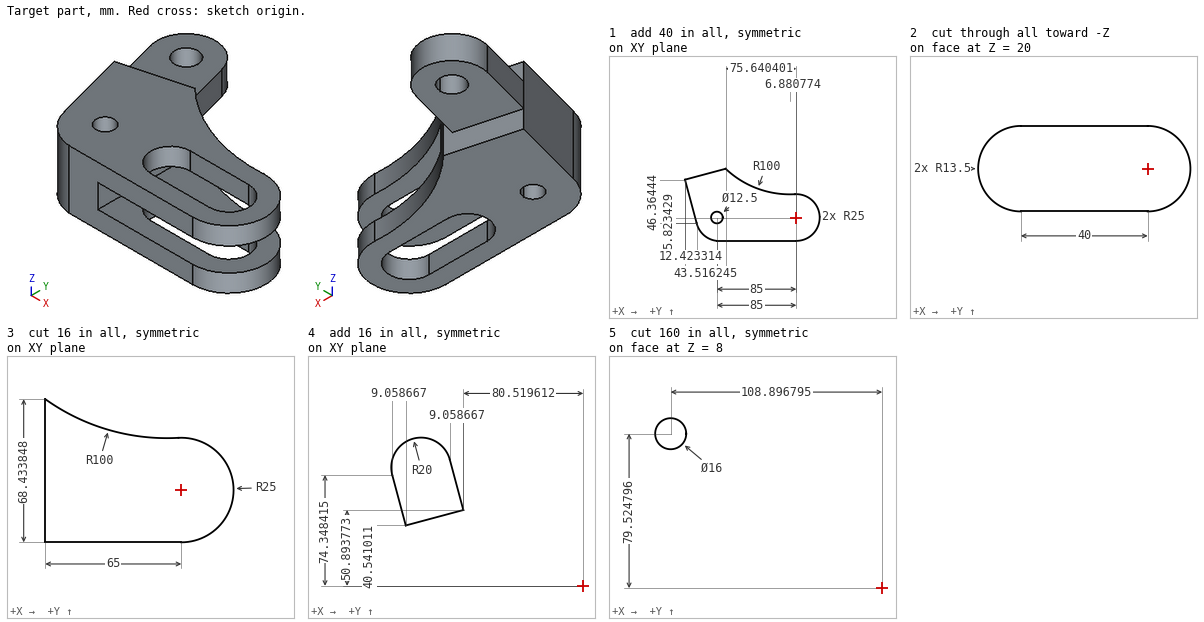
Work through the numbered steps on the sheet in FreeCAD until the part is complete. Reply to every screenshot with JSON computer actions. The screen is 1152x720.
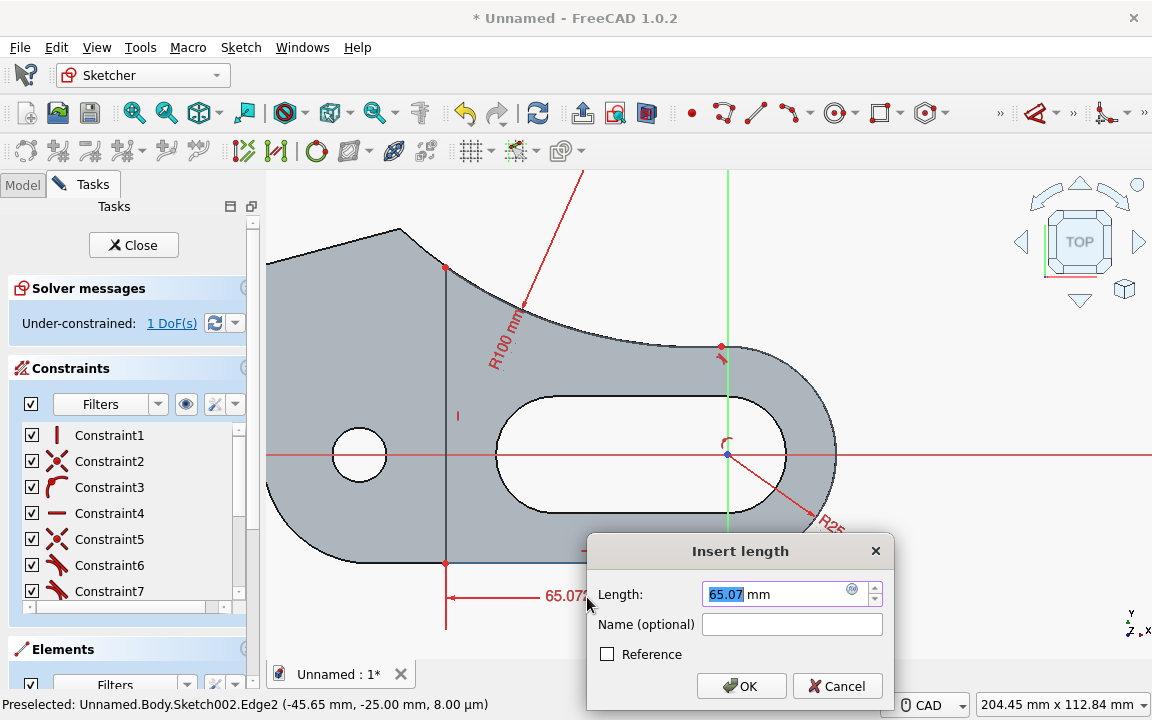
{"action": "type", "text": "65"}
{"action": "key", "text": "Return"}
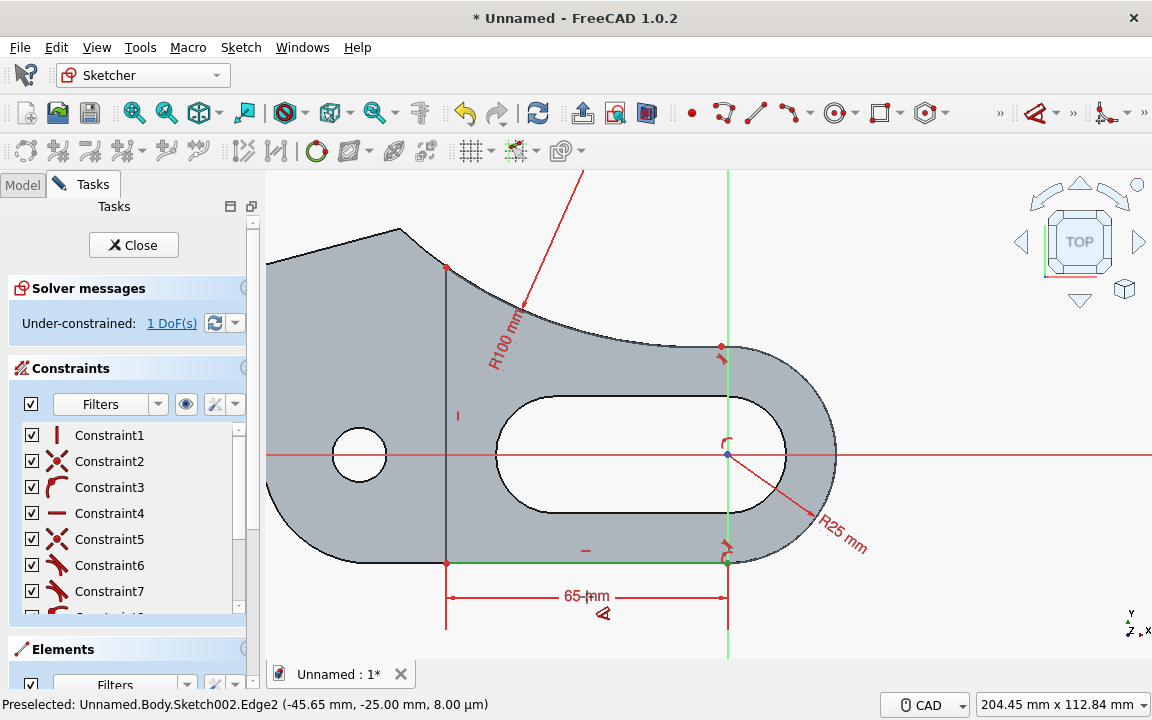
{"action": "left_click", "coordinate": [446, 356]}
{"action": "left_click", "coordinate": [412, 415]}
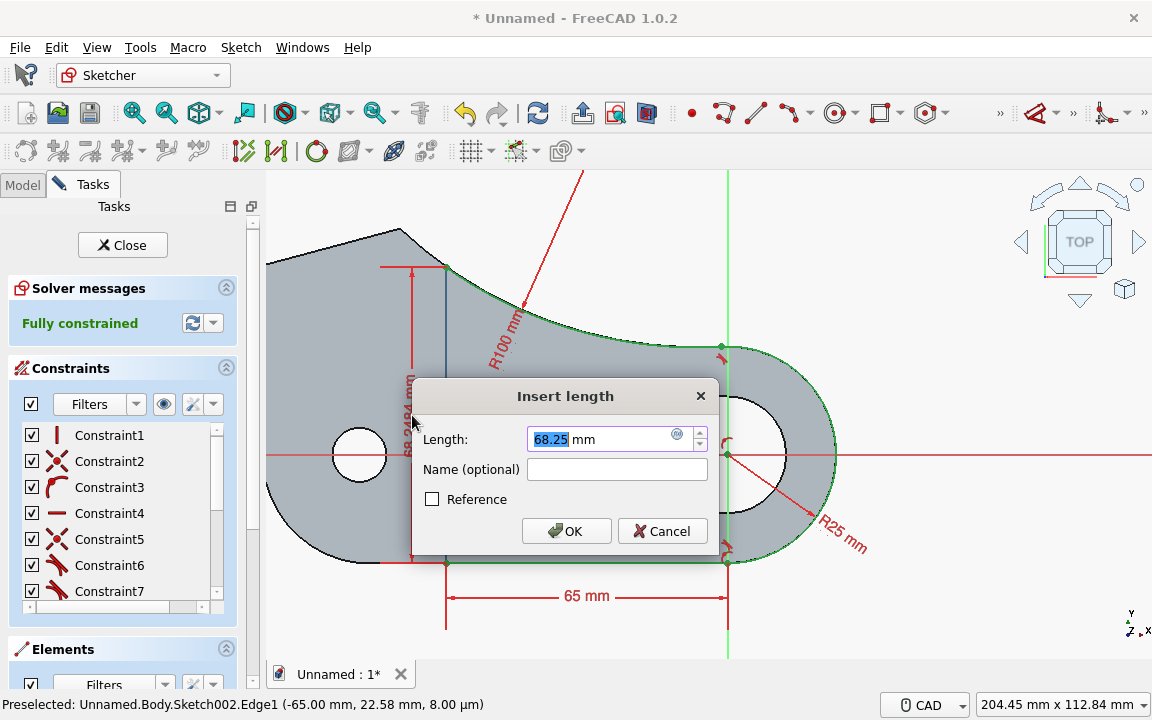
{"action": "type", "text": "68.433848"}
{"action": "key", "text": "Return"}
{"action": "key", "text": "Escape"}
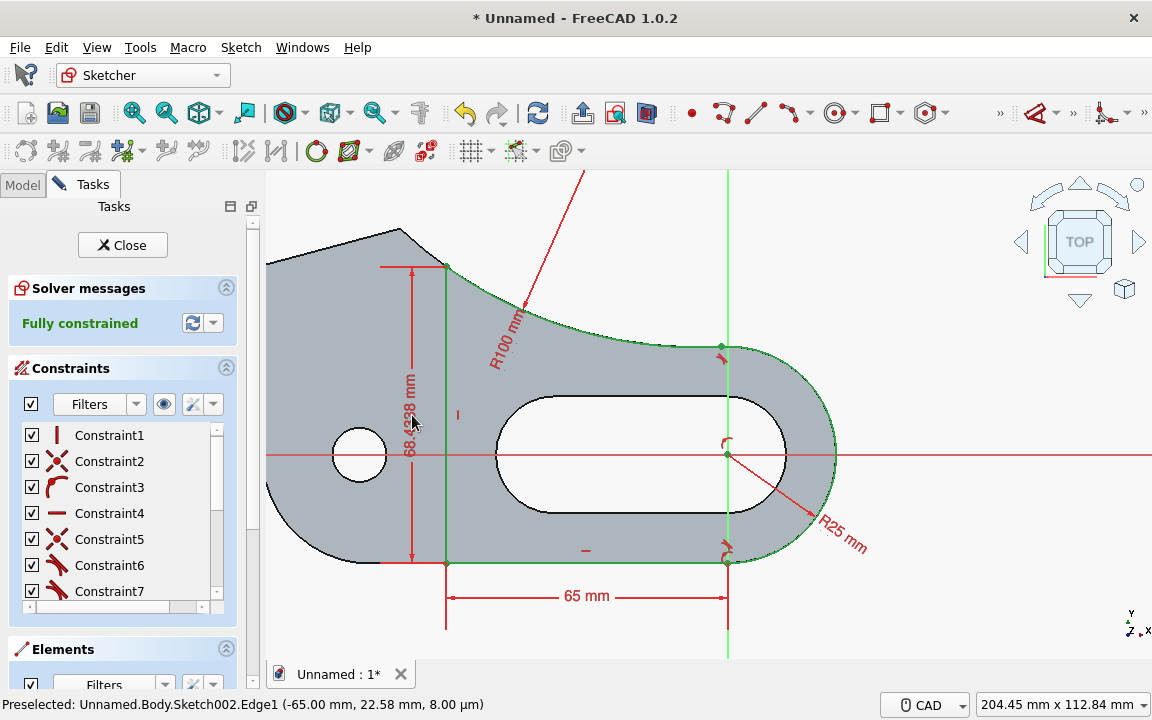
{"action": "left_click", "coordinate": [123, 245]}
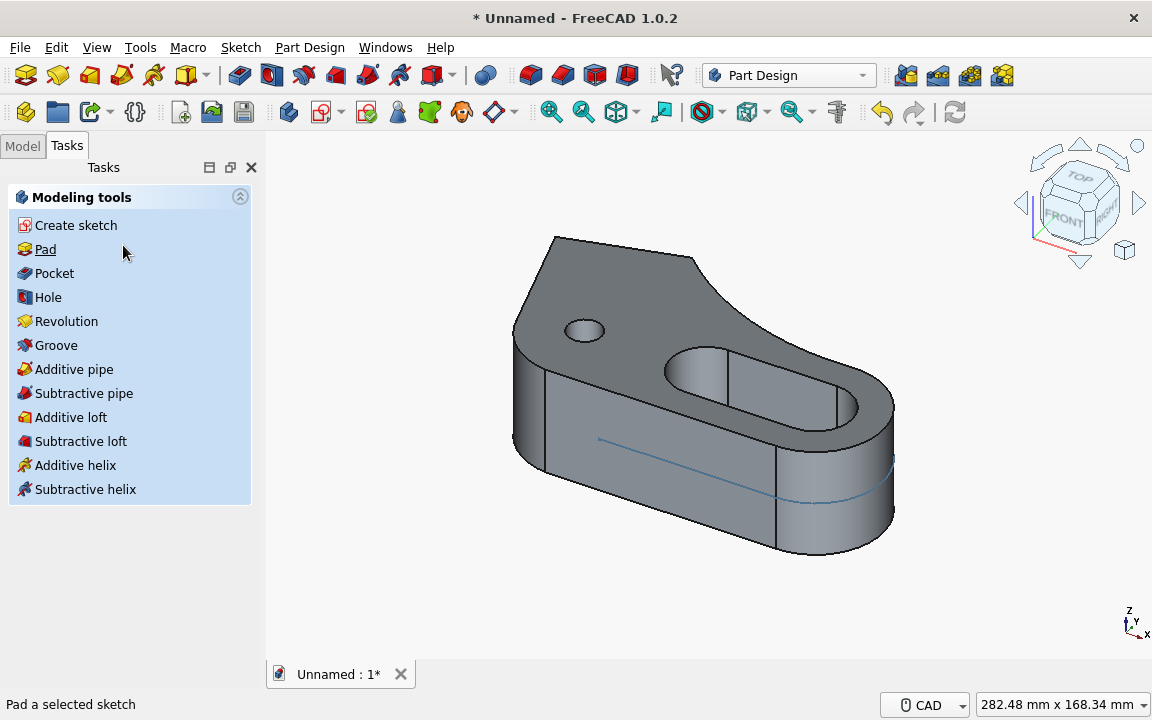
{"action": "left_click", "coordinate": [240, 76]}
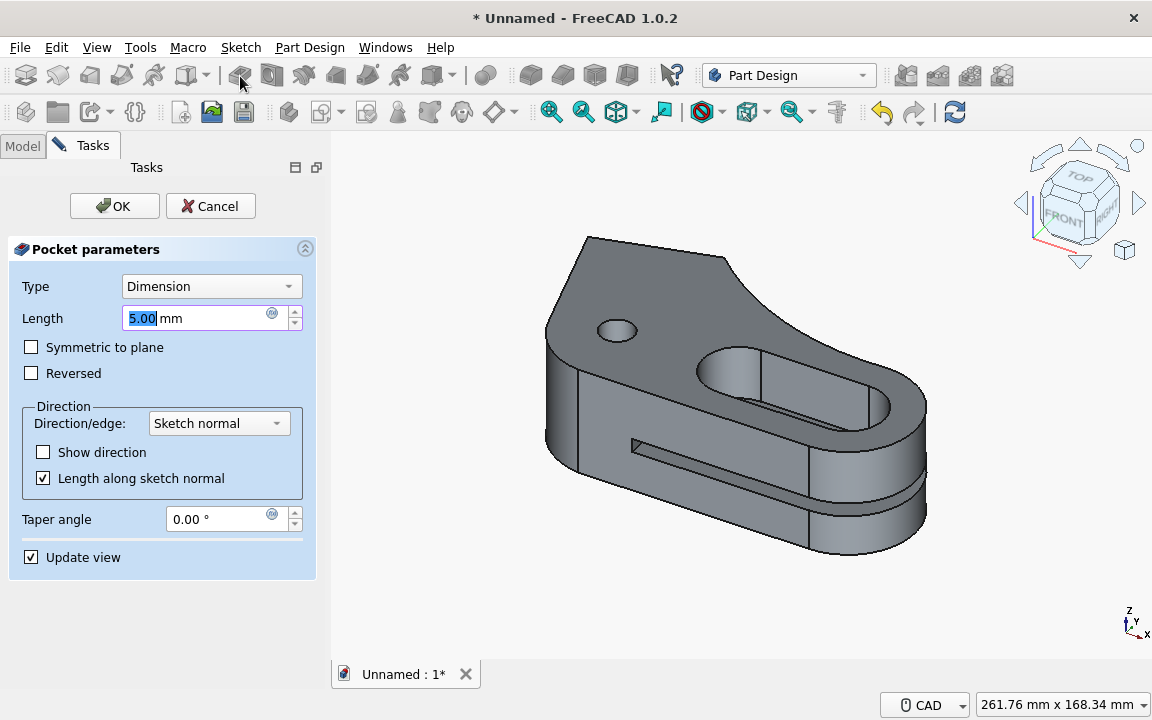
{"action": "type", "text": "16"}
{"action": "key", "text": "Tab"}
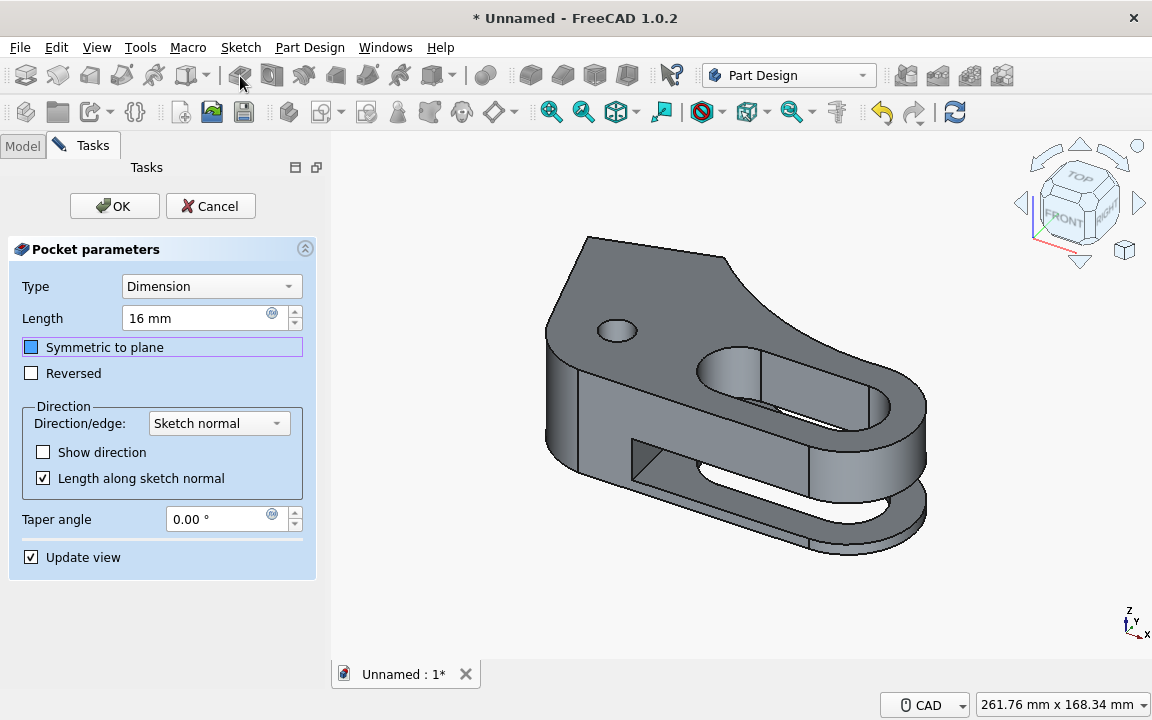
{"action": "left_click", "coordinate": [30, 347]}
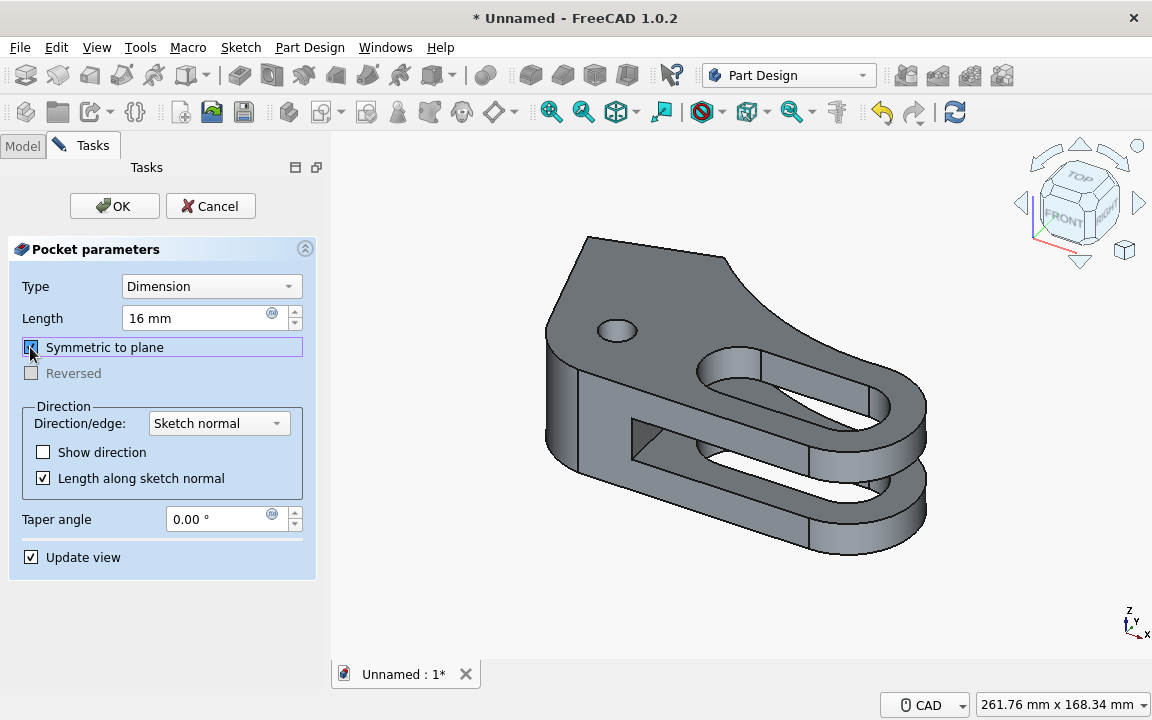
{"action": "left_click", "coordinate": [115, 206]}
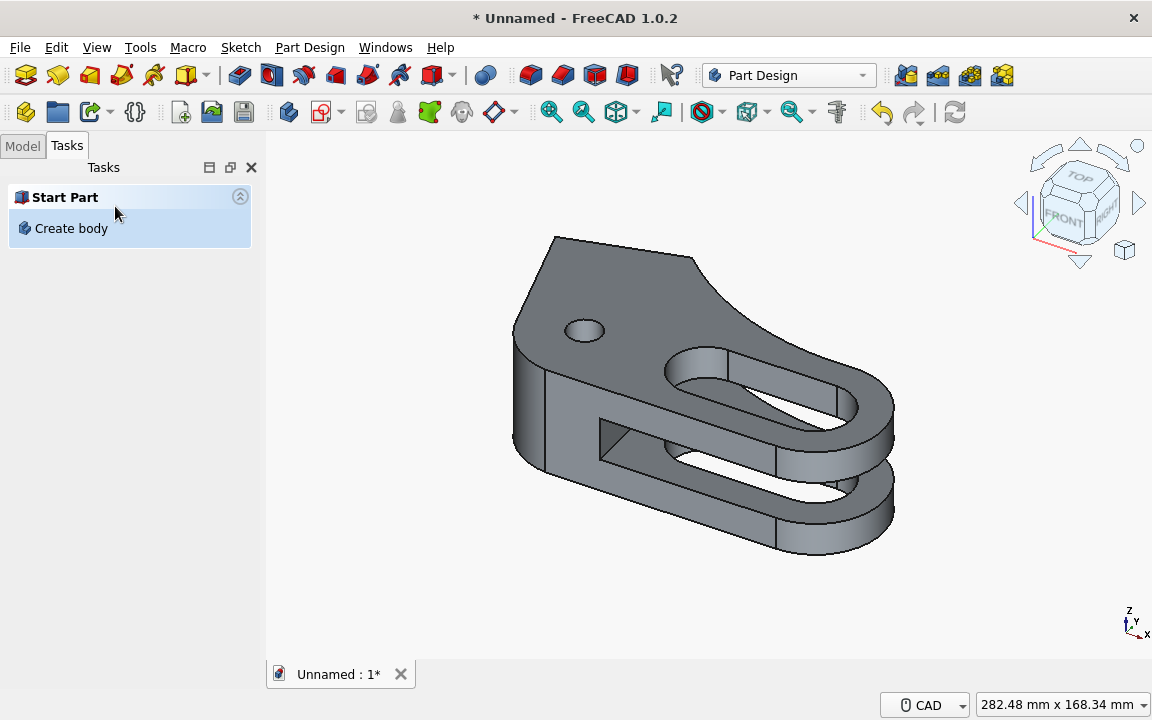
{"action": "left_click", "coordinate": [322, 112]}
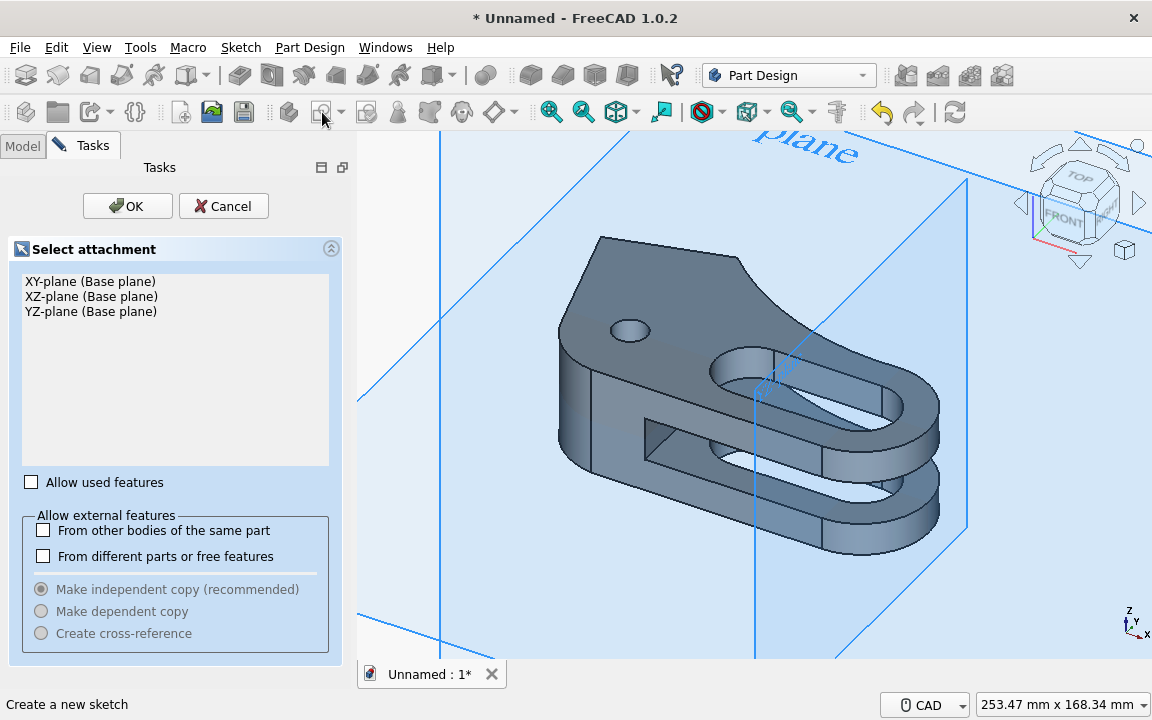
{"action": "left_click", "coordinate": [82, 282]}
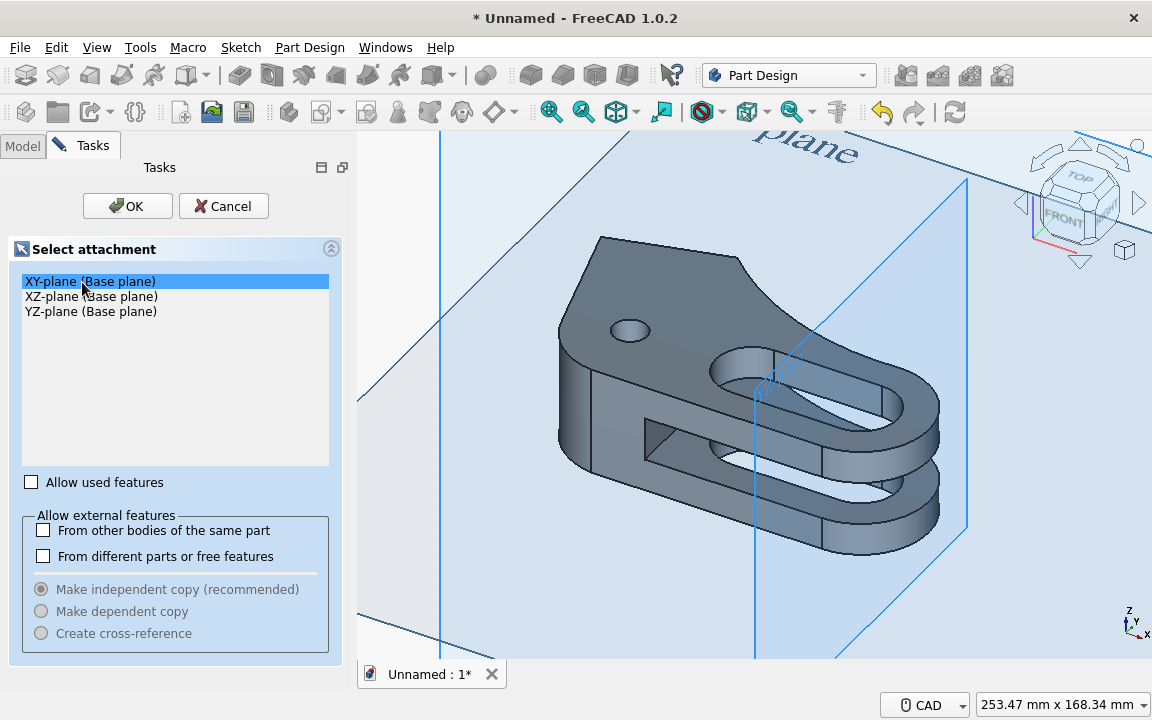
{"action": "left_click", "coordinate": [128, 206]}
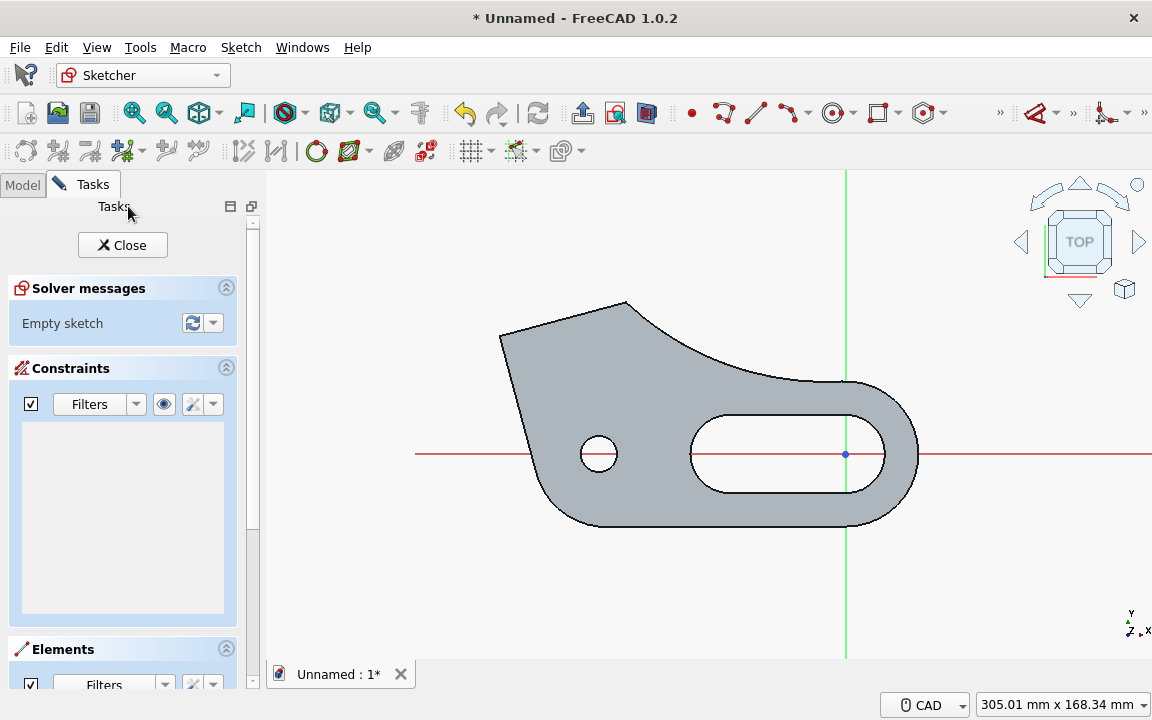
{"action": "left_click", "coordinate": [648, 114]}